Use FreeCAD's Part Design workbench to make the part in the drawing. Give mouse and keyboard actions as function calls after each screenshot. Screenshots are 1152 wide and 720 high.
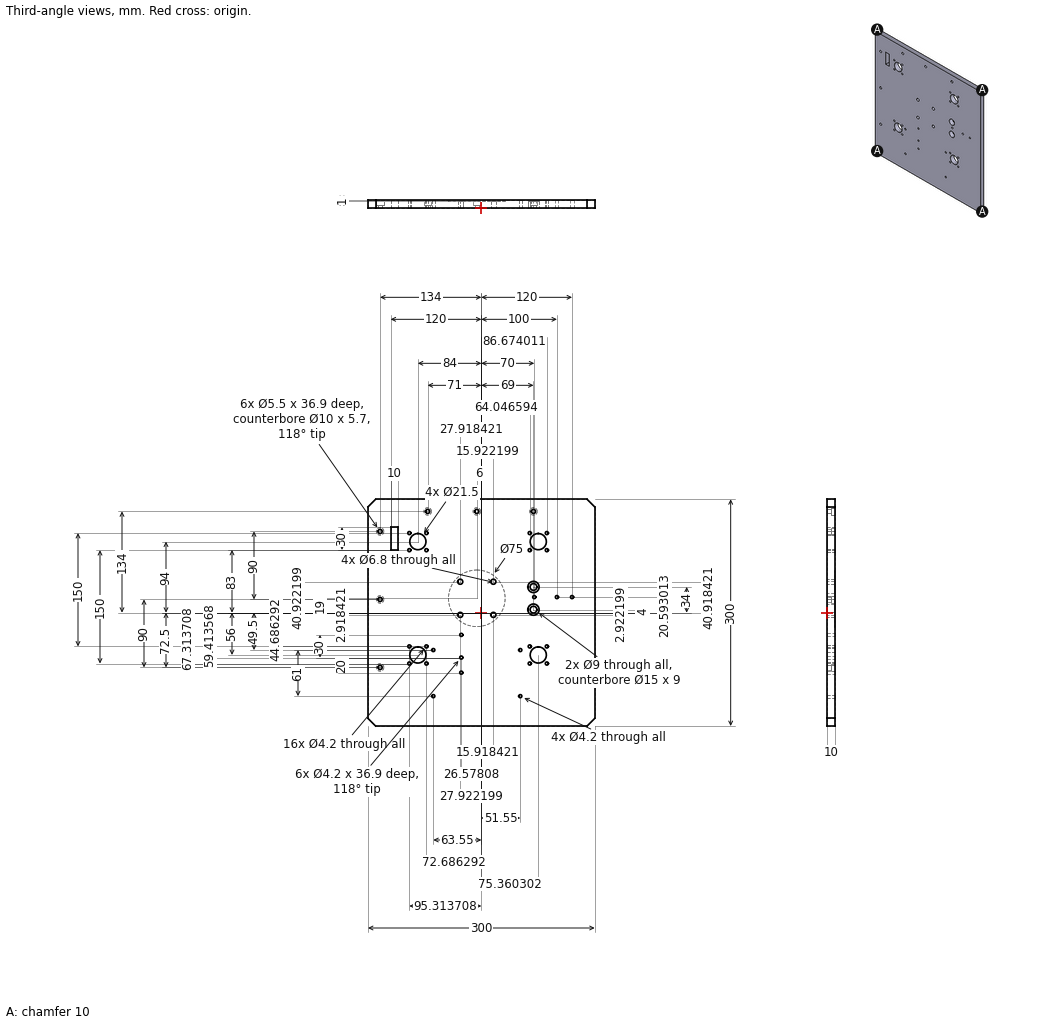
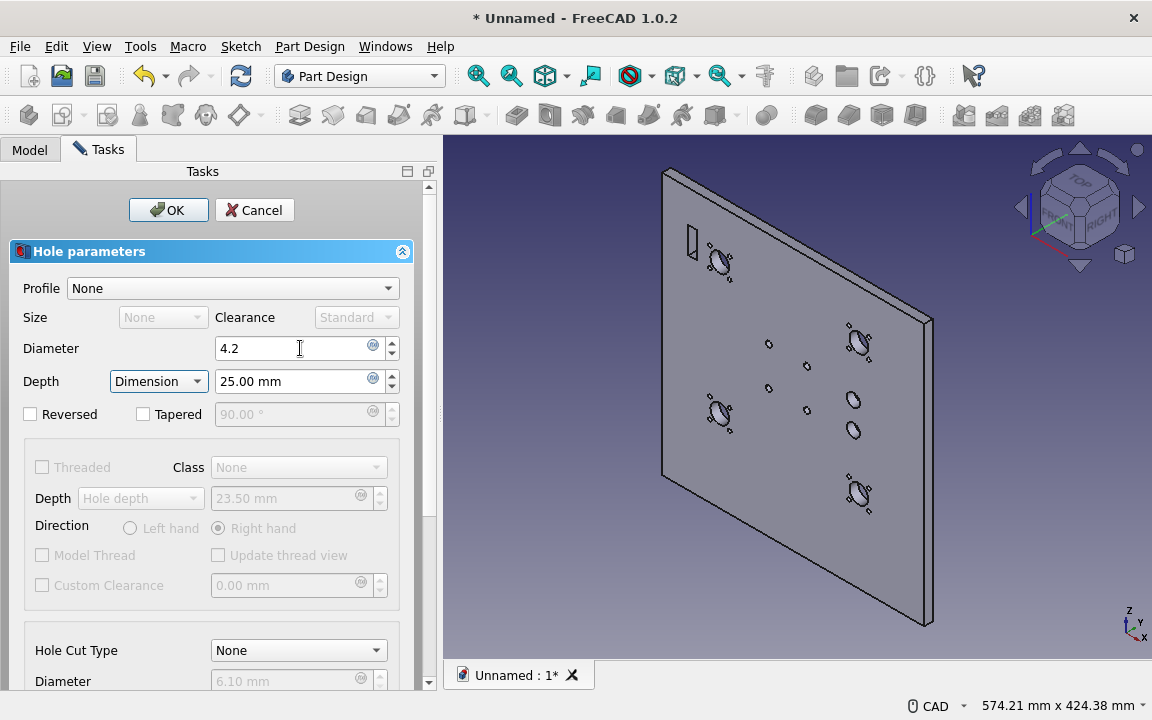
click(160, 382)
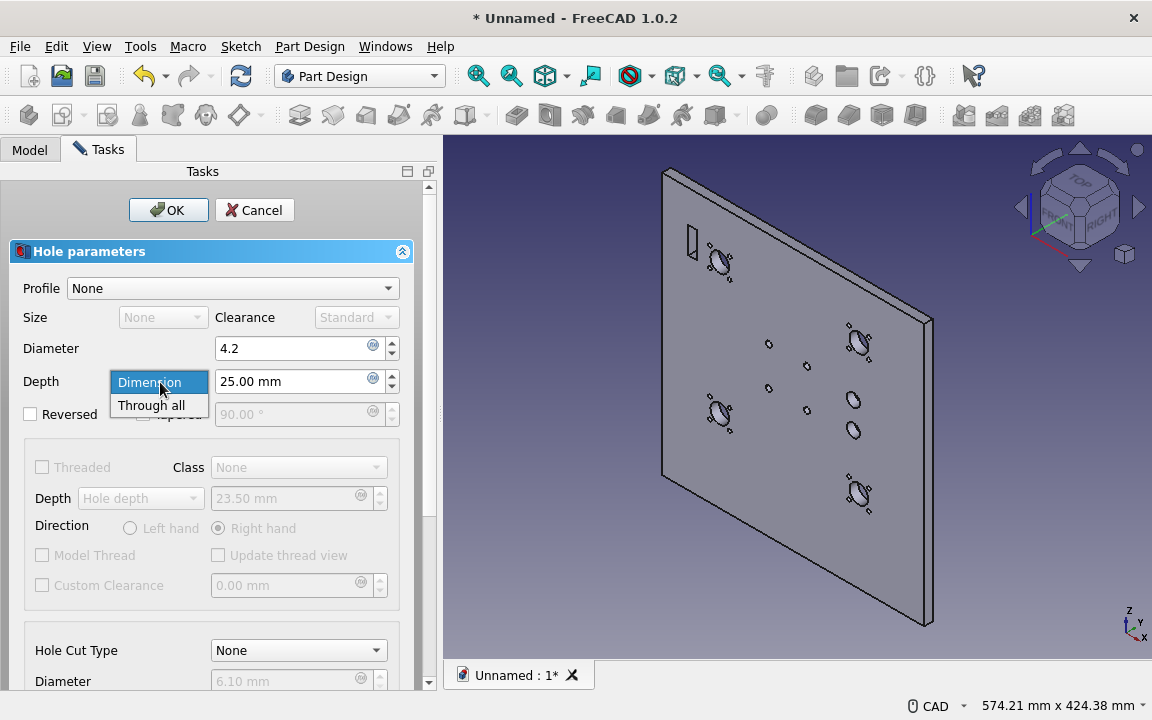
click(158, 406)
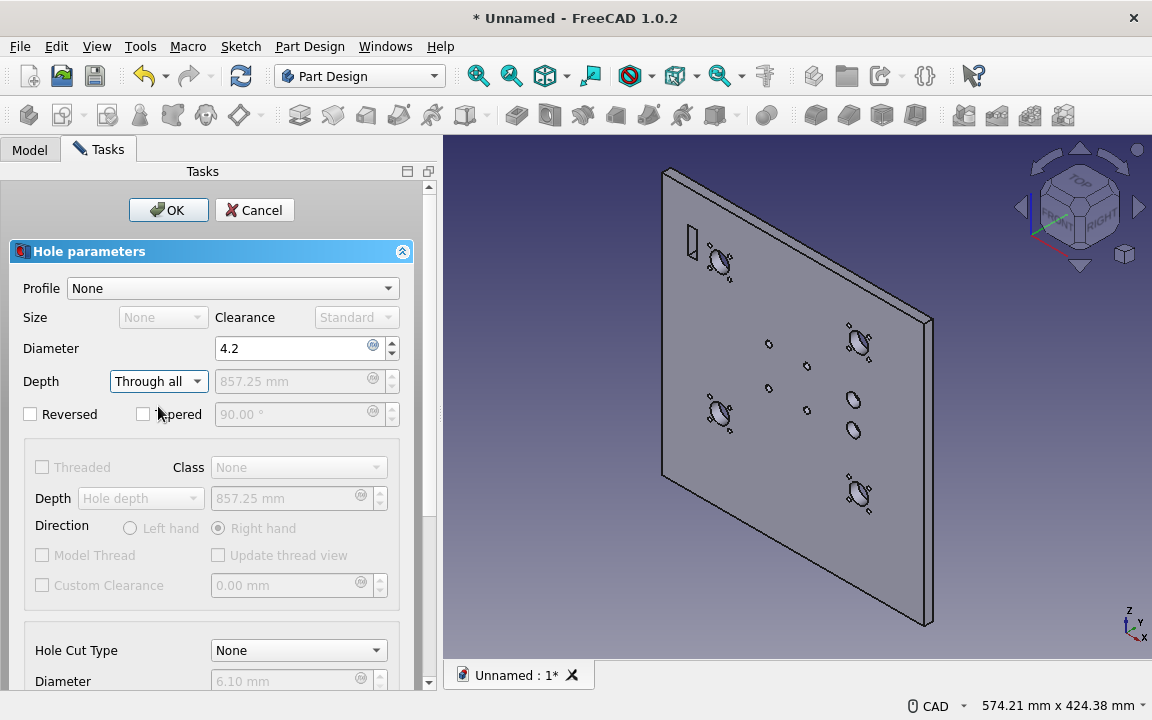
click(169, 210)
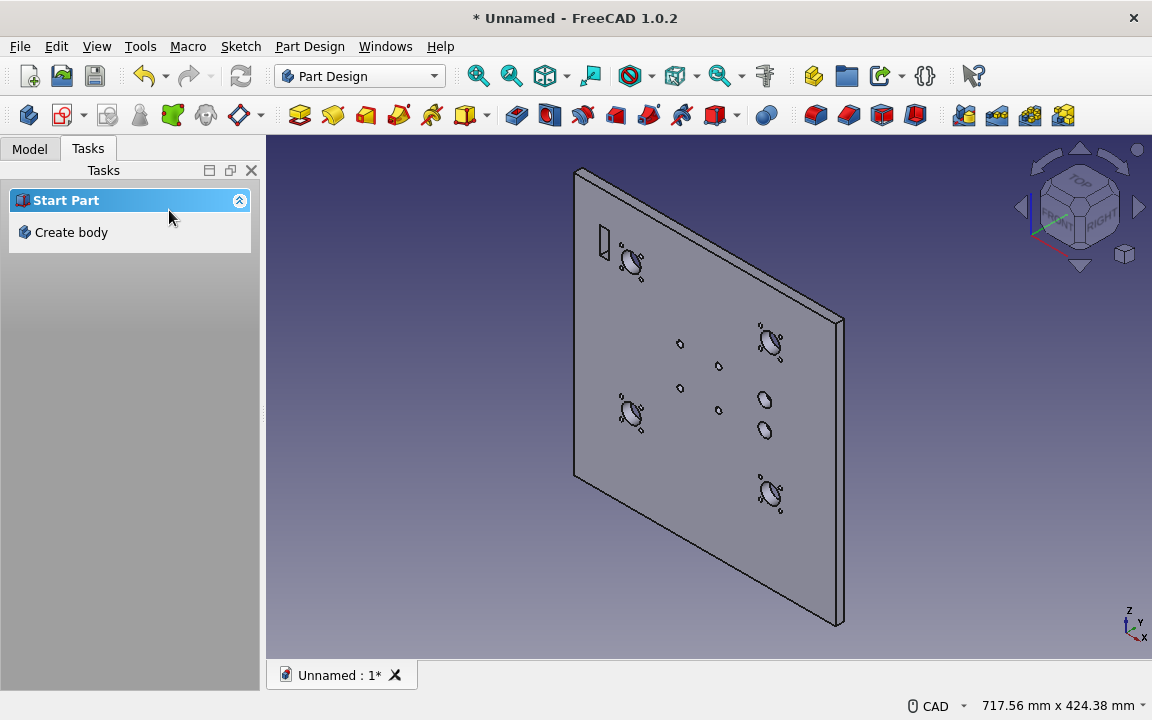
key(4)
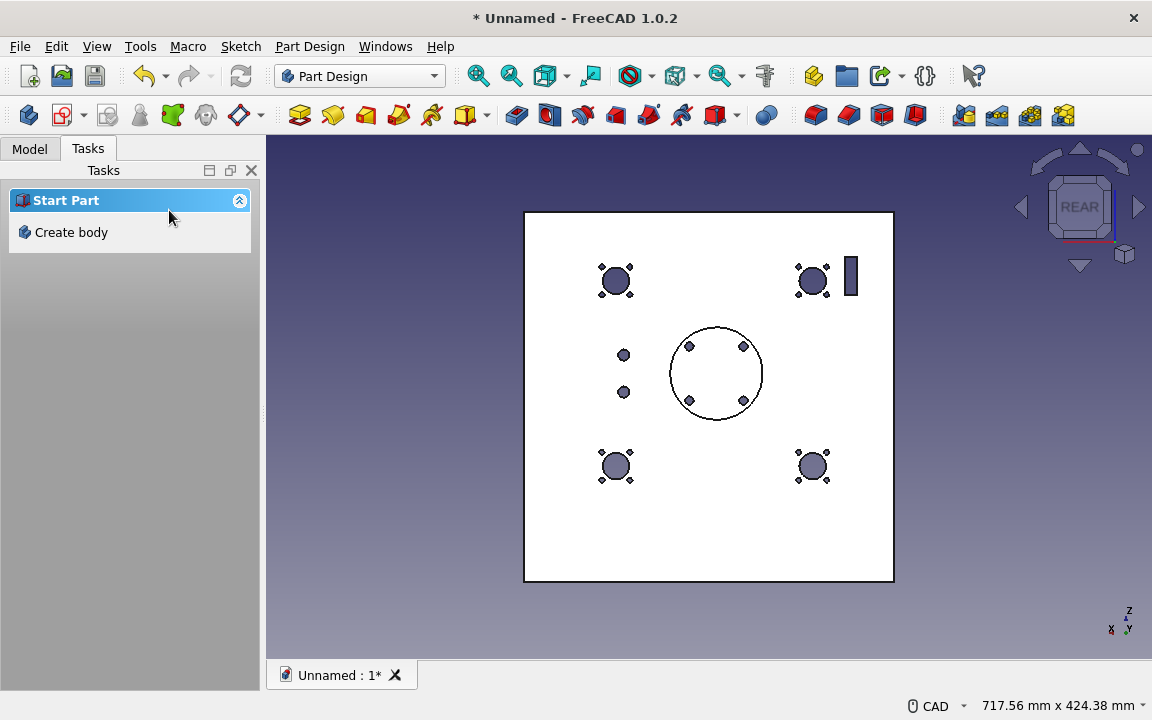
click(709, 502)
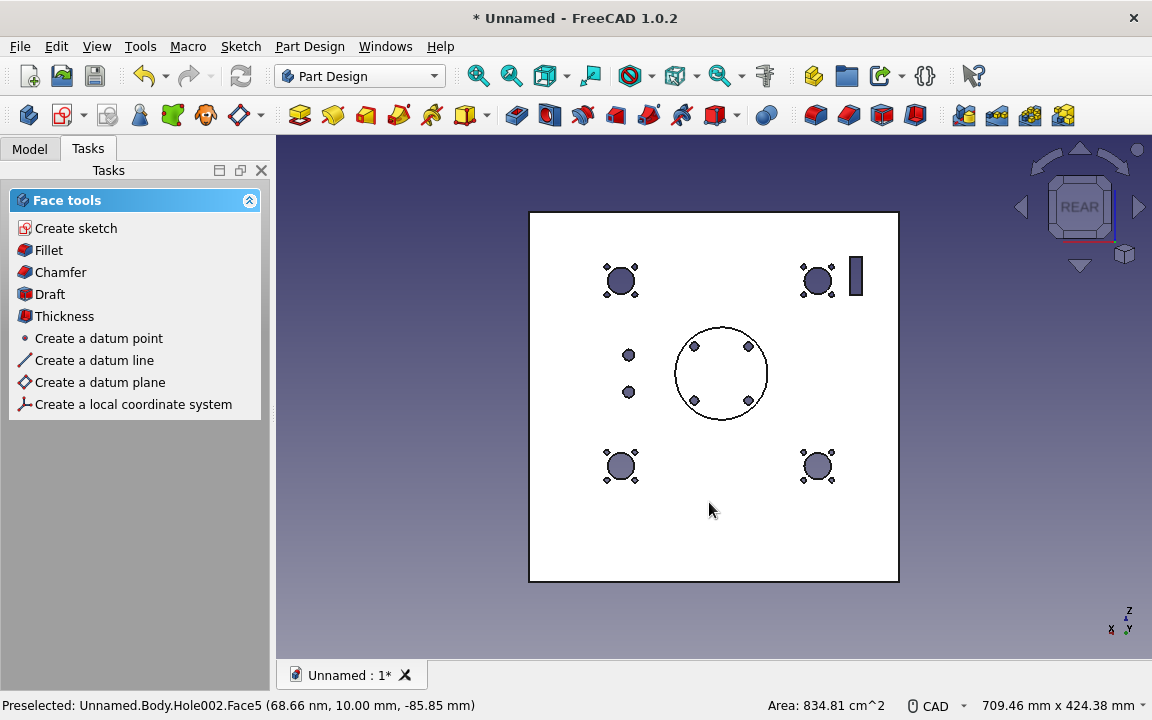
click(62, 116)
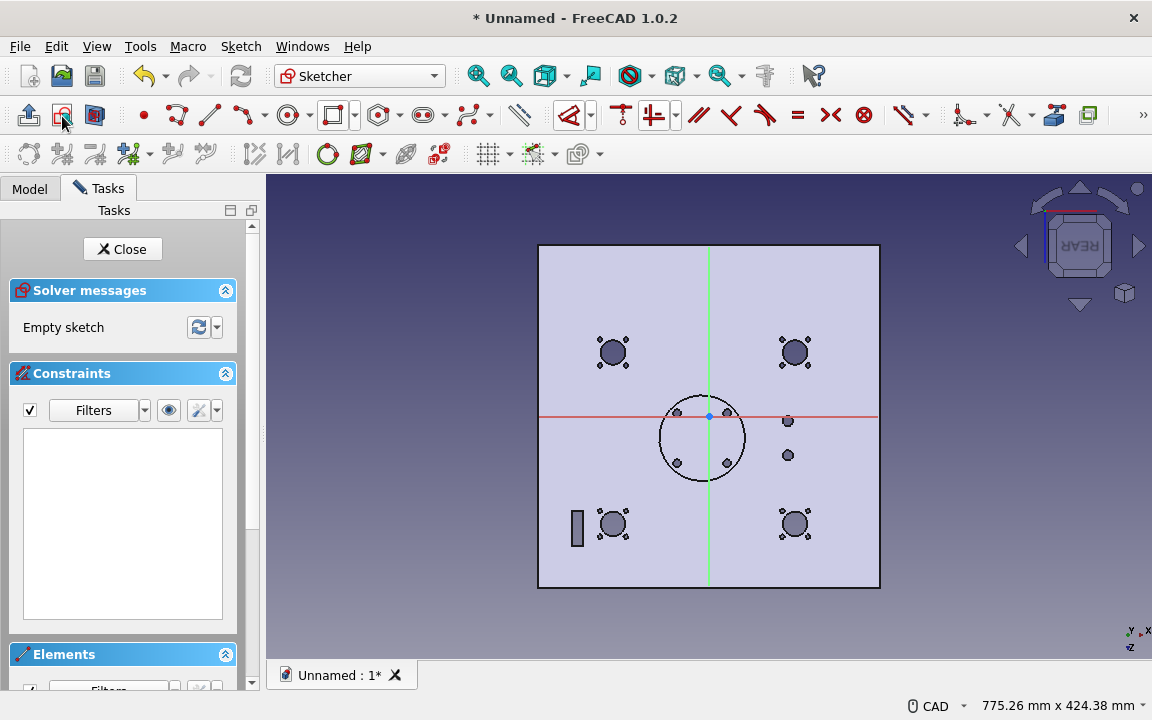
scroll(752, 300, up, 4)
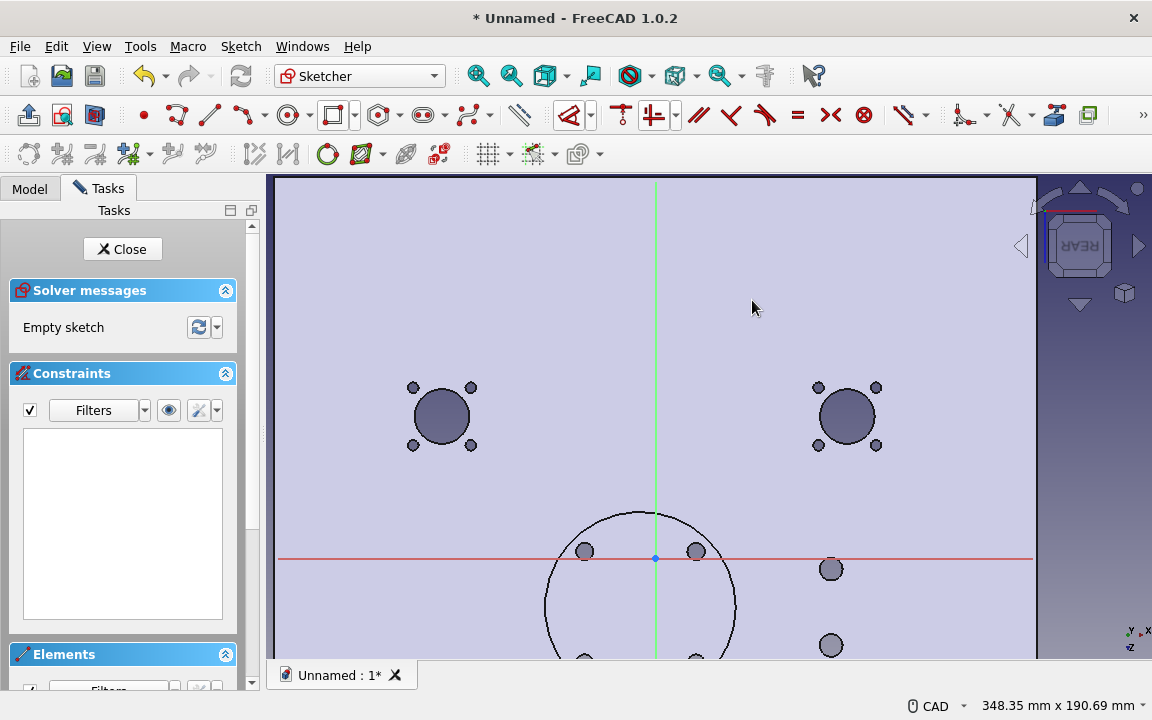
click(288, 116)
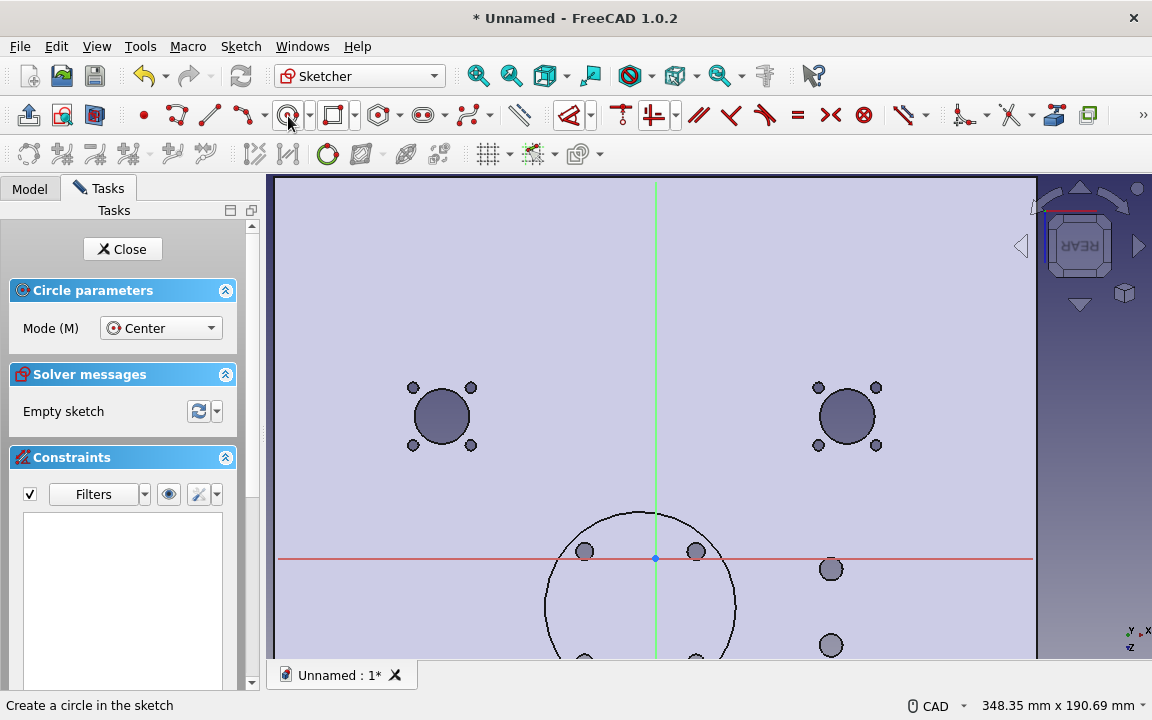
scroll(787, 278, up, 8)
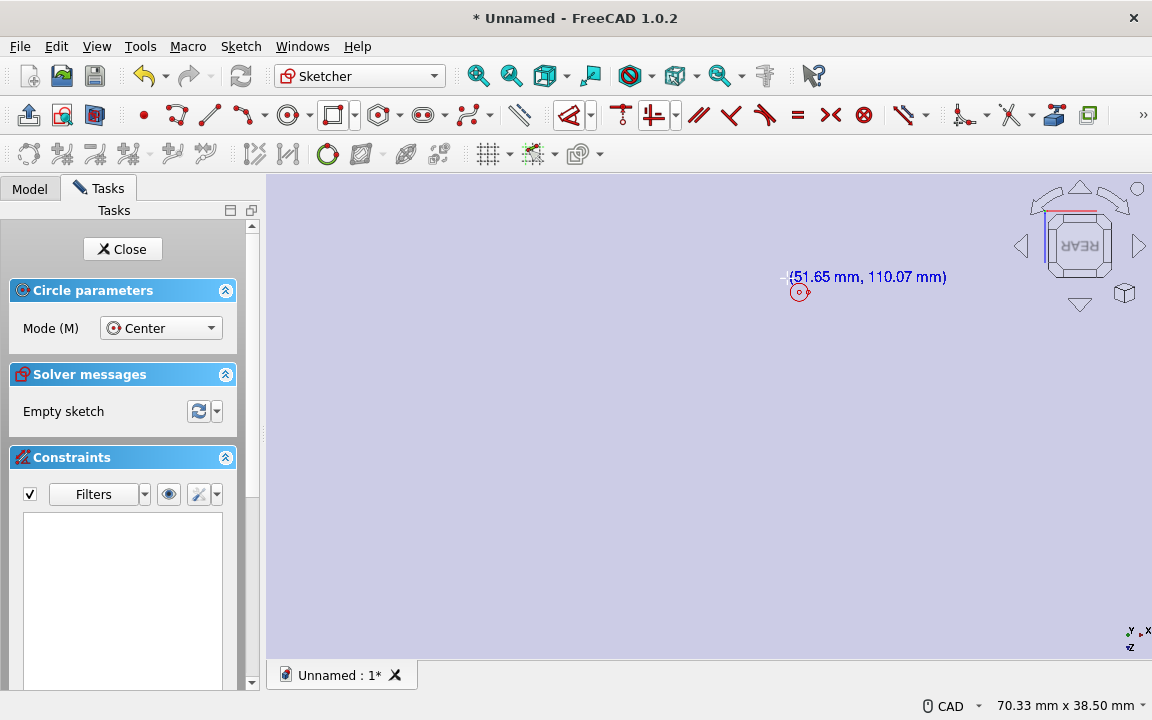
scroll(788, 279, down, 8)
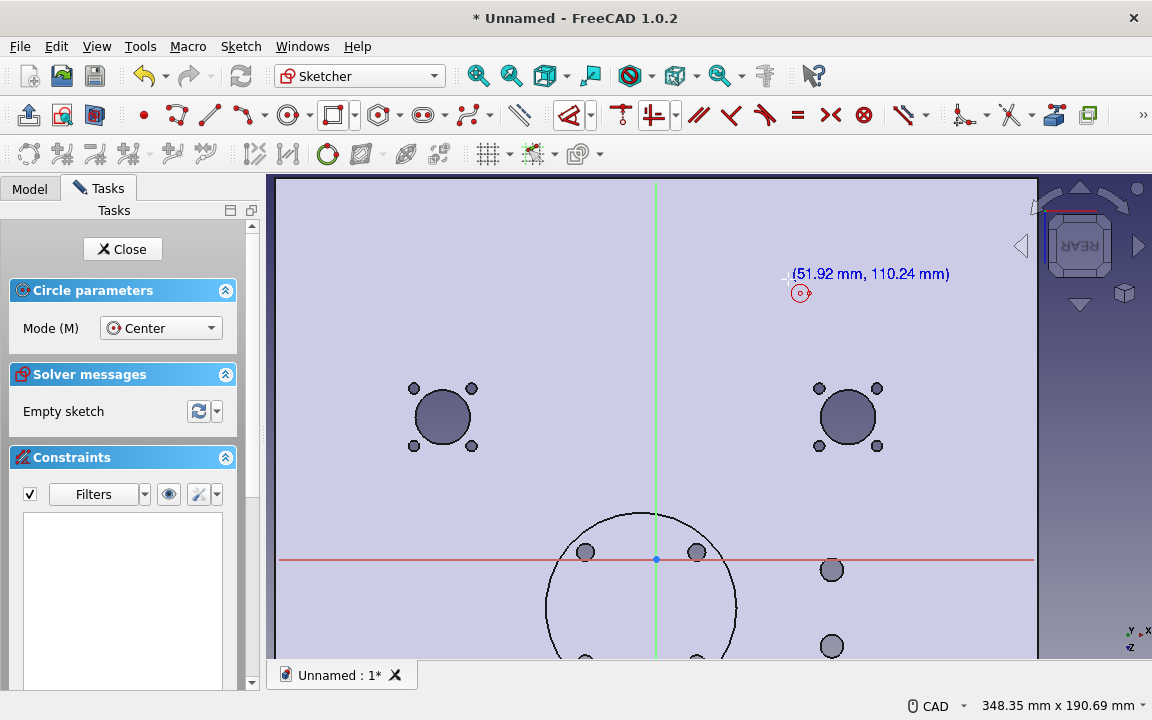
click(788, 279)
move(791, 275)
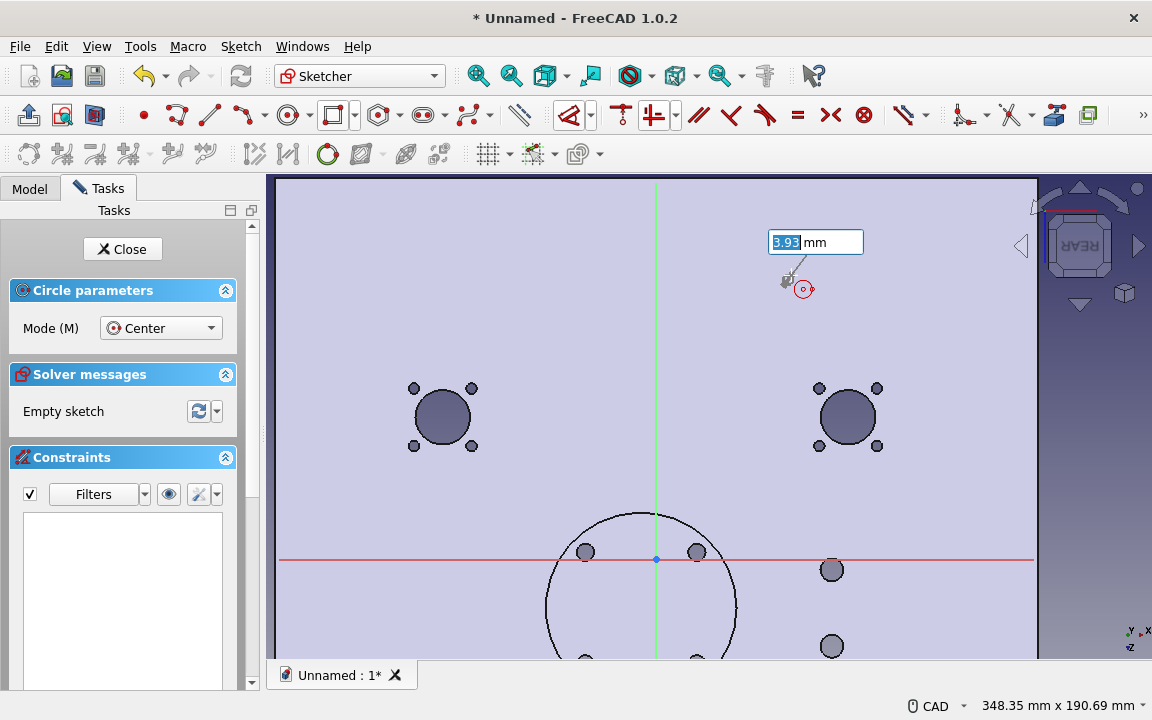
text(4.2)
key(Return)